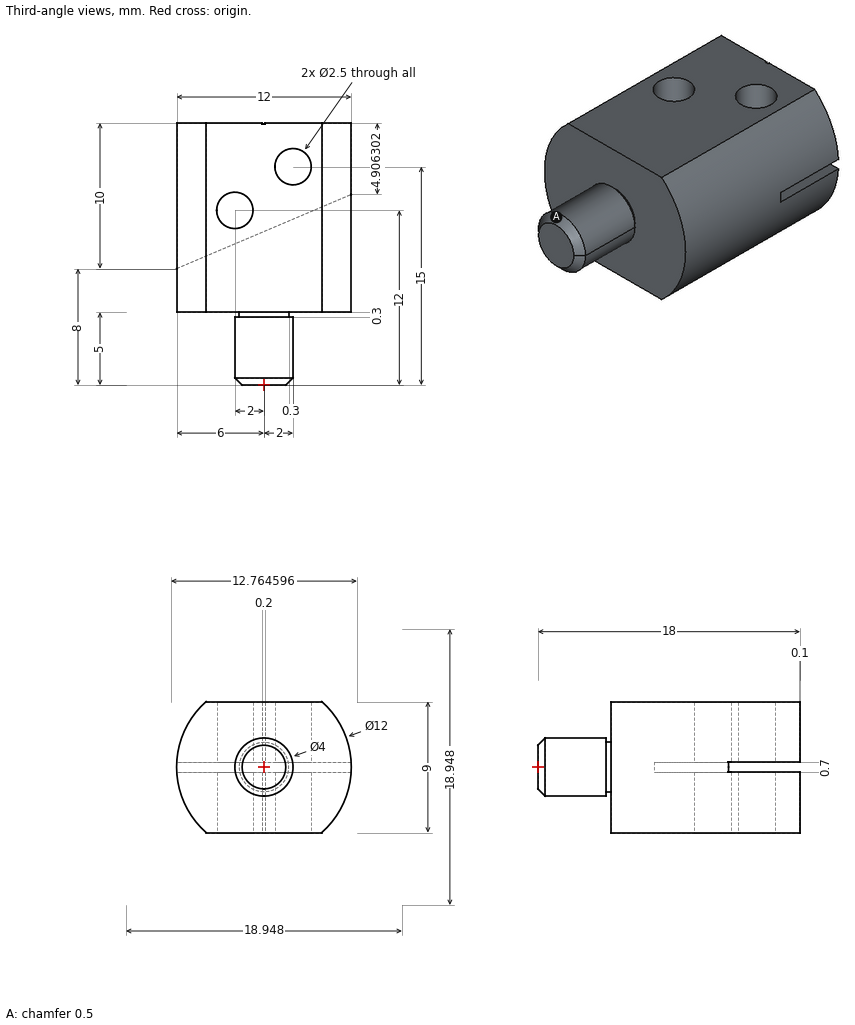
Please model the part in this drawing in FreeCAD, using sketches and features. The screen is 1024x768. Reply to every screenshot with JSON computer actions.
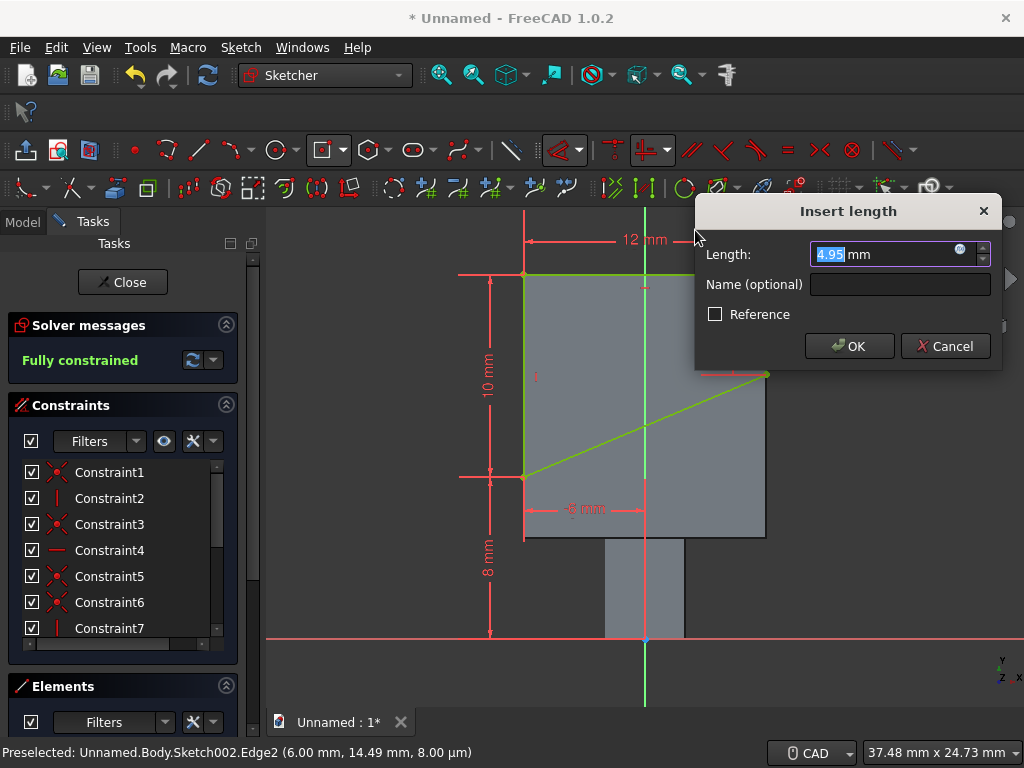
{"action": "type", "text": "4.906302"}
{"action": "key", "text": "Return"}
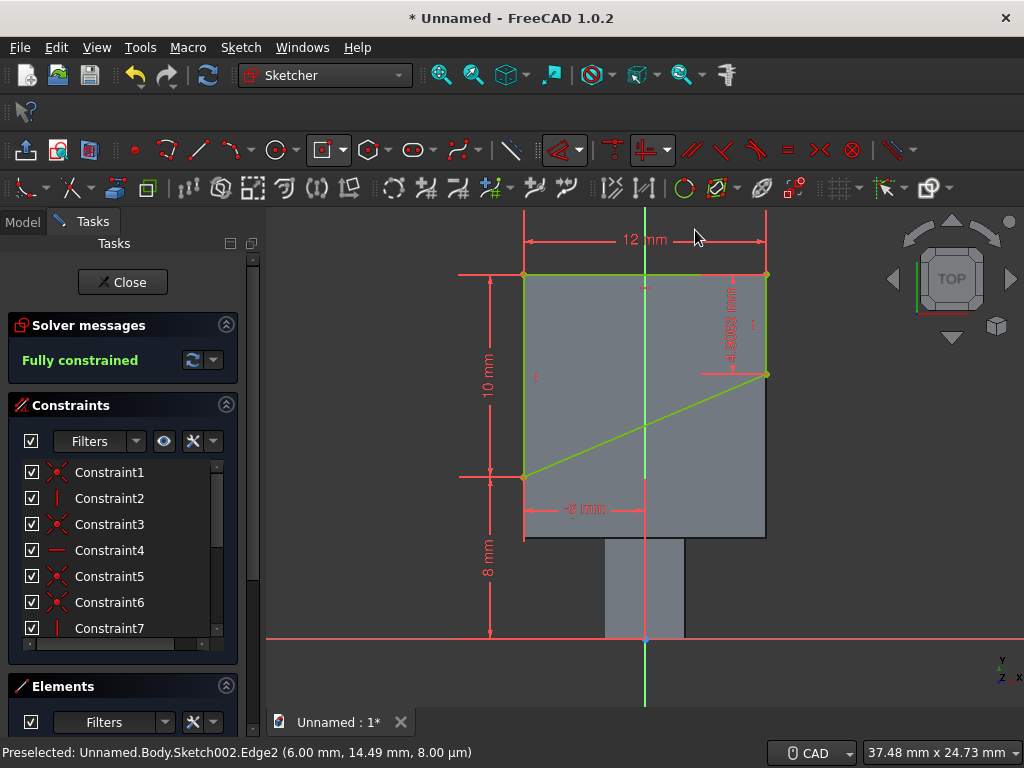
{"action": "left_click", "coordinate": [123, 282]}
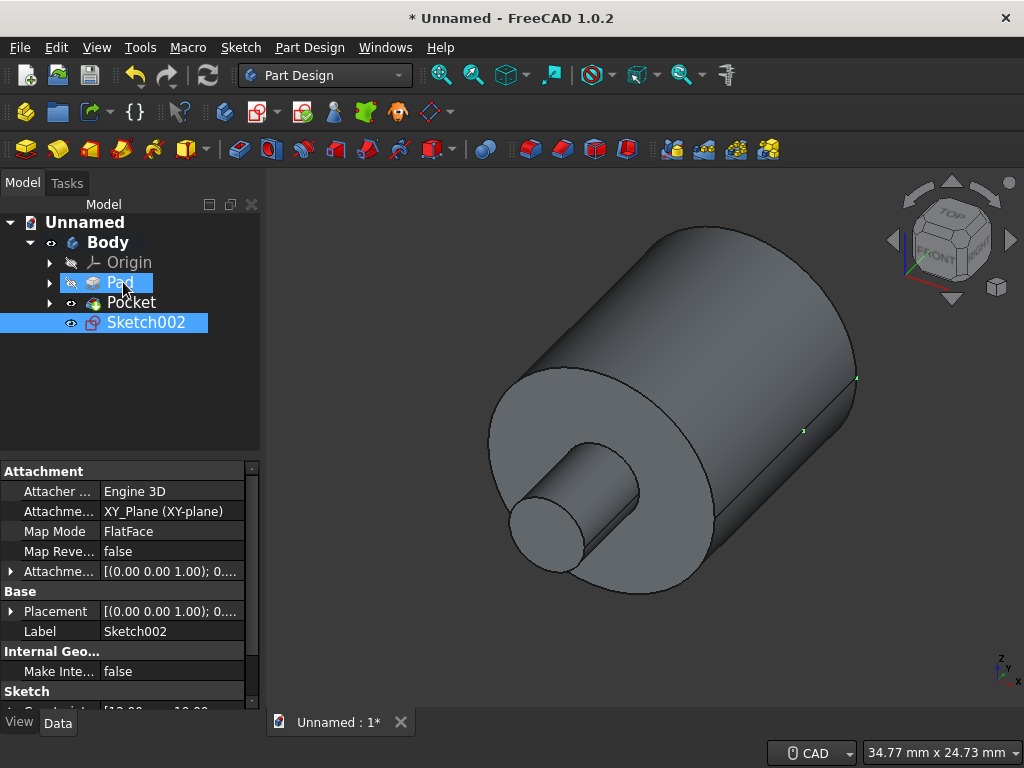
{"action": "left_click", "coordinate": [240, 150]}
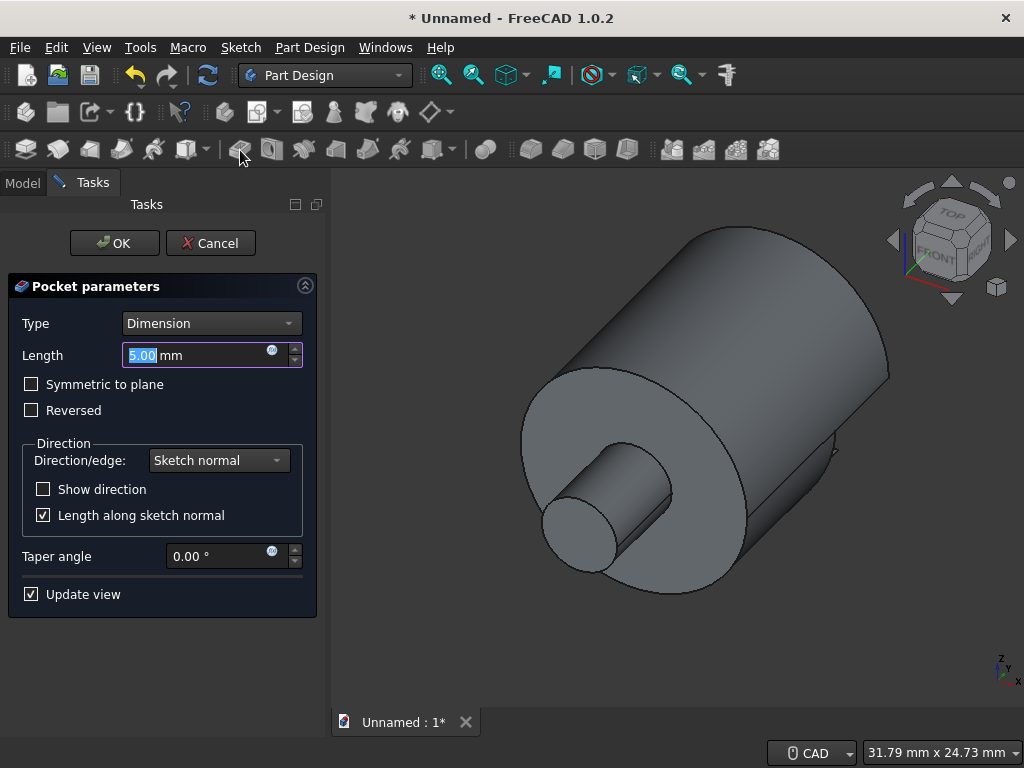
{"action": "type", "text": "0.7"}
{"action": "key", "text": "Tab"}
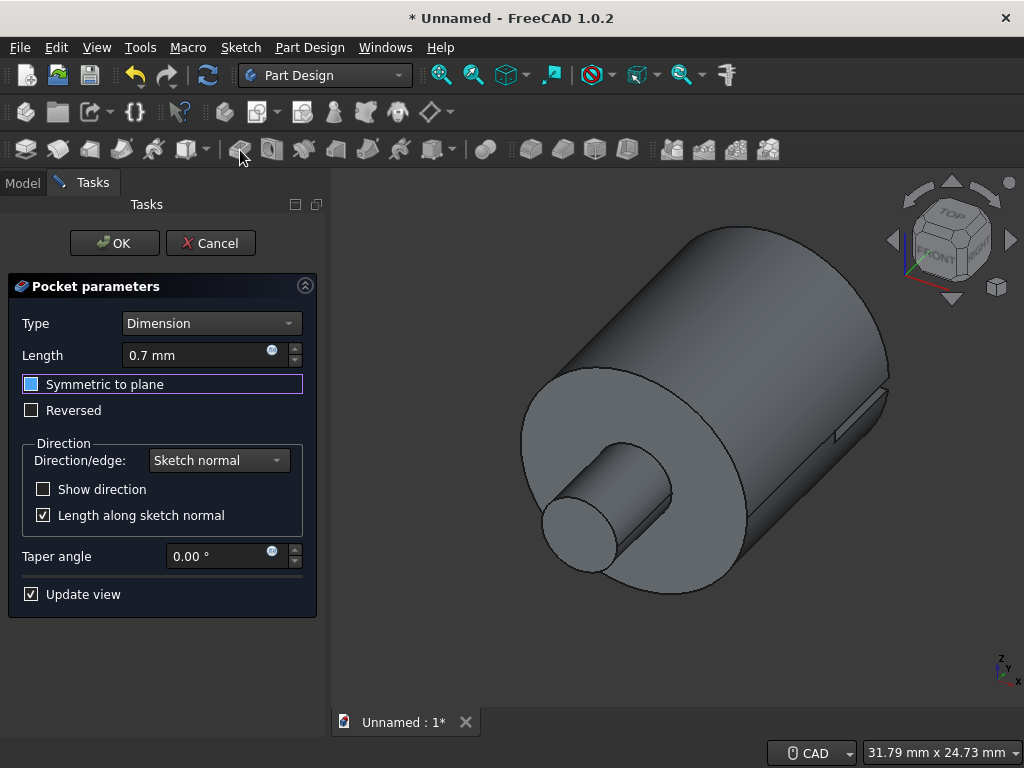
{"action": "left_click", "coordinate": [30, 384]}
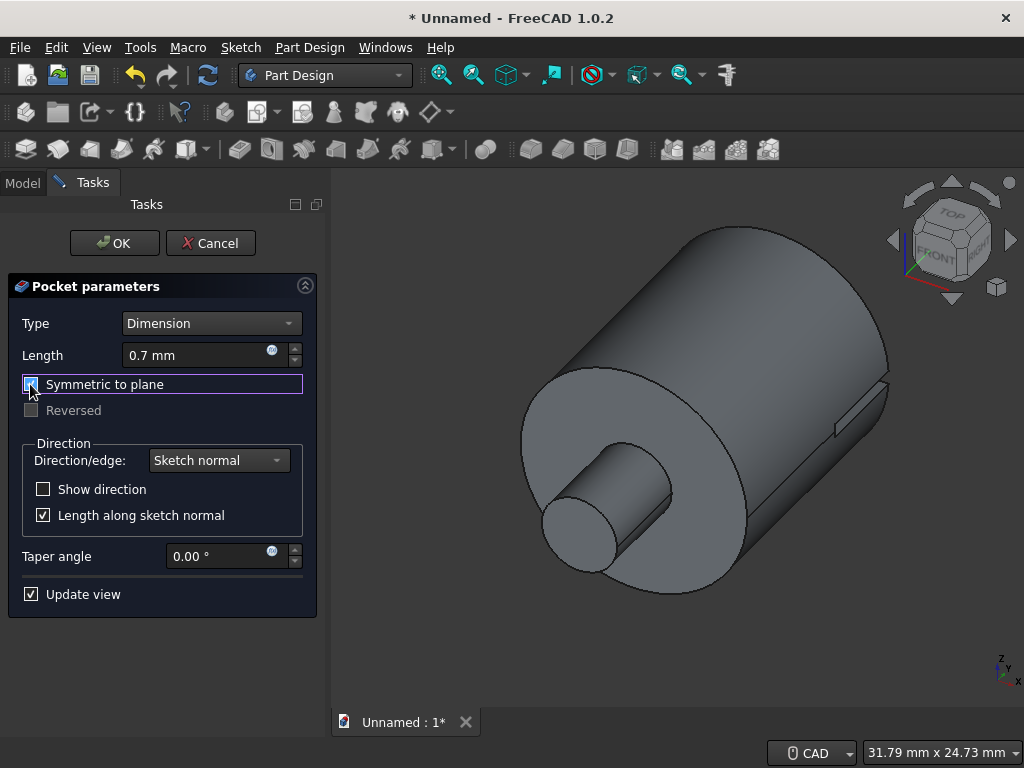
{"action": "left_click", "coordinate": [115, 243]}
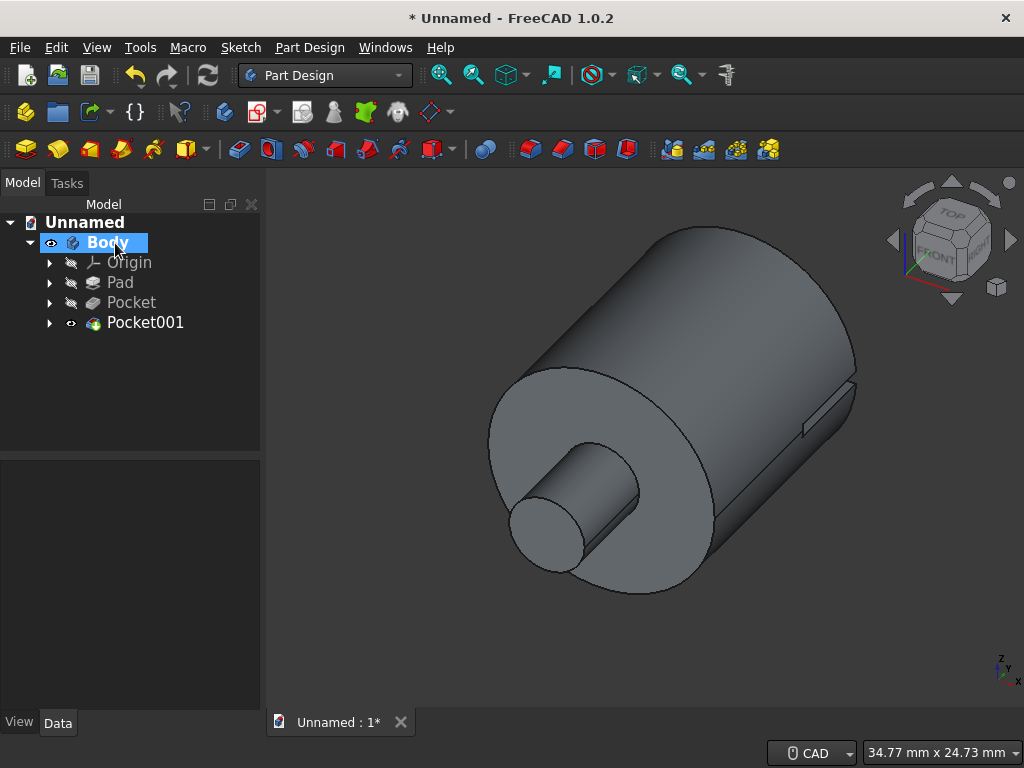
{"action": "left_click", "coordinate": [516, 503]}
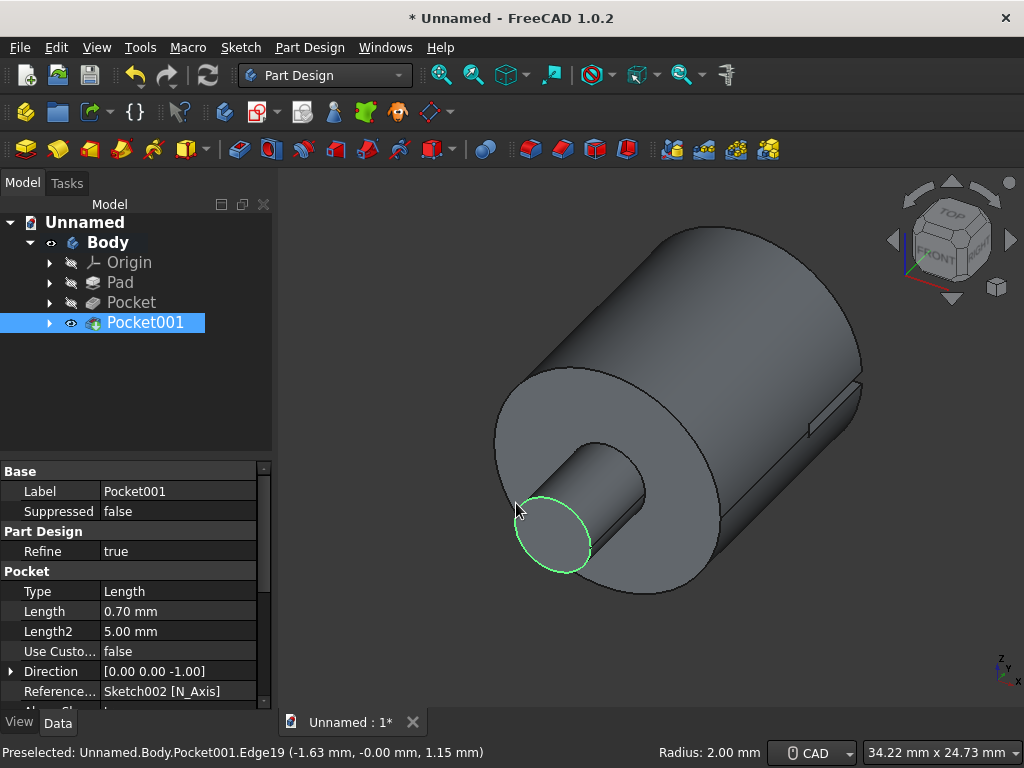
{"action": "left_click", "coordinate": [564, 150]}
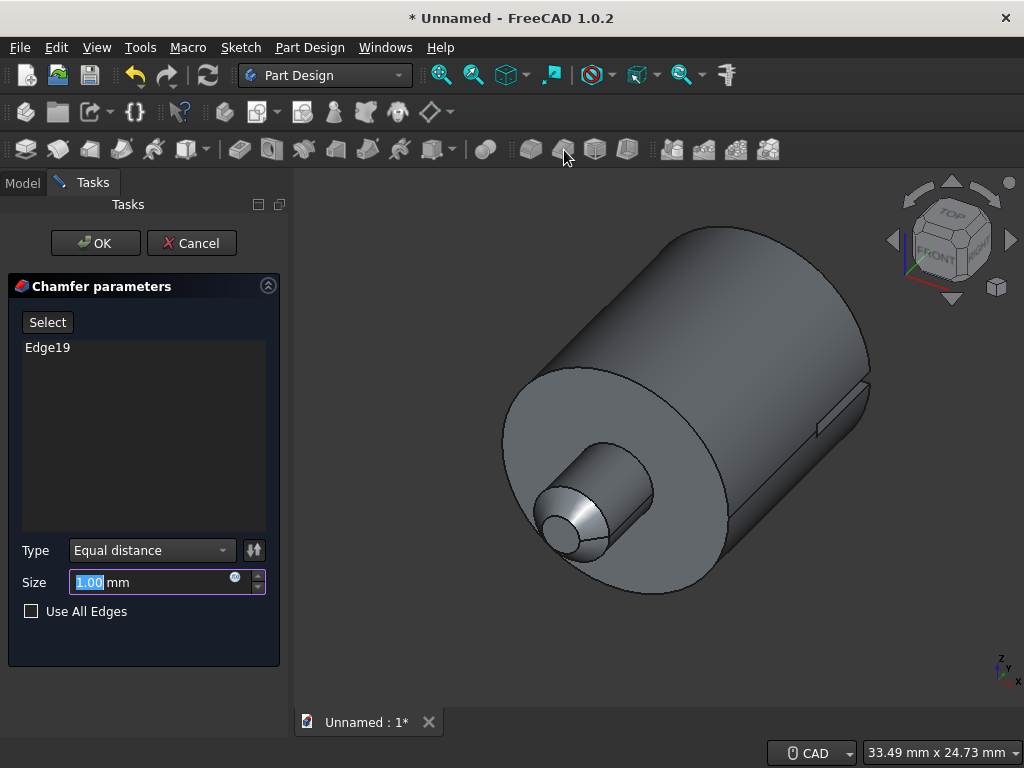
{"action": "type", "text": "0.5"}
{"action": "key", "text": "Tab"}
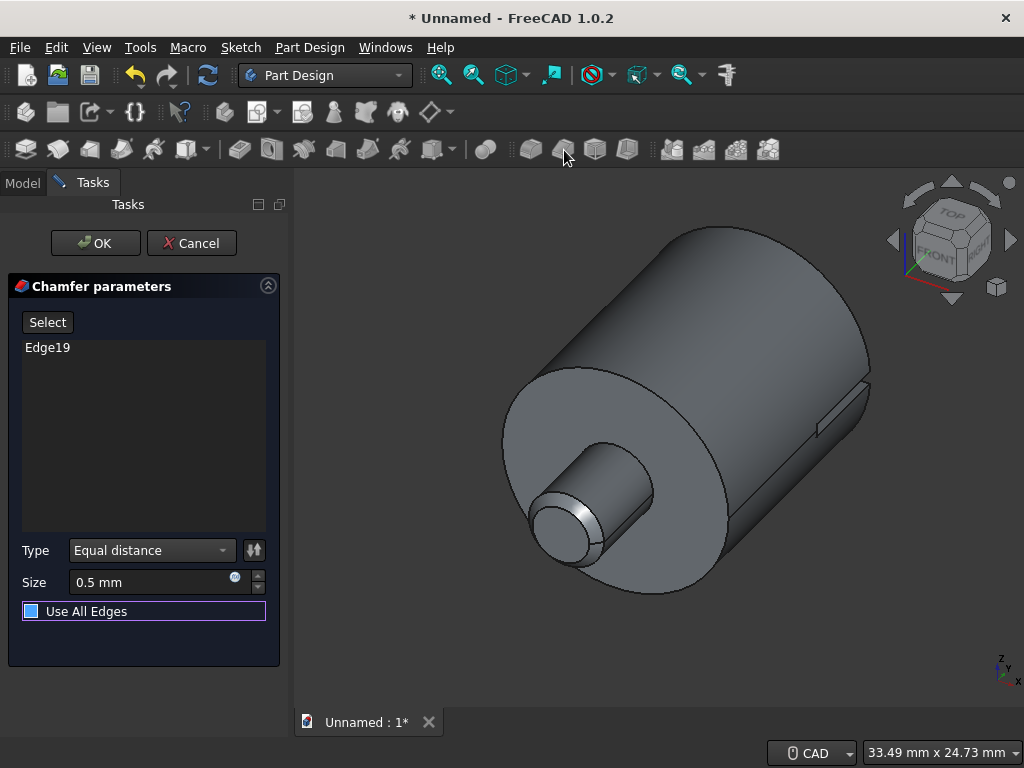
{"action": "left_click", "coordinate": [96, 243]}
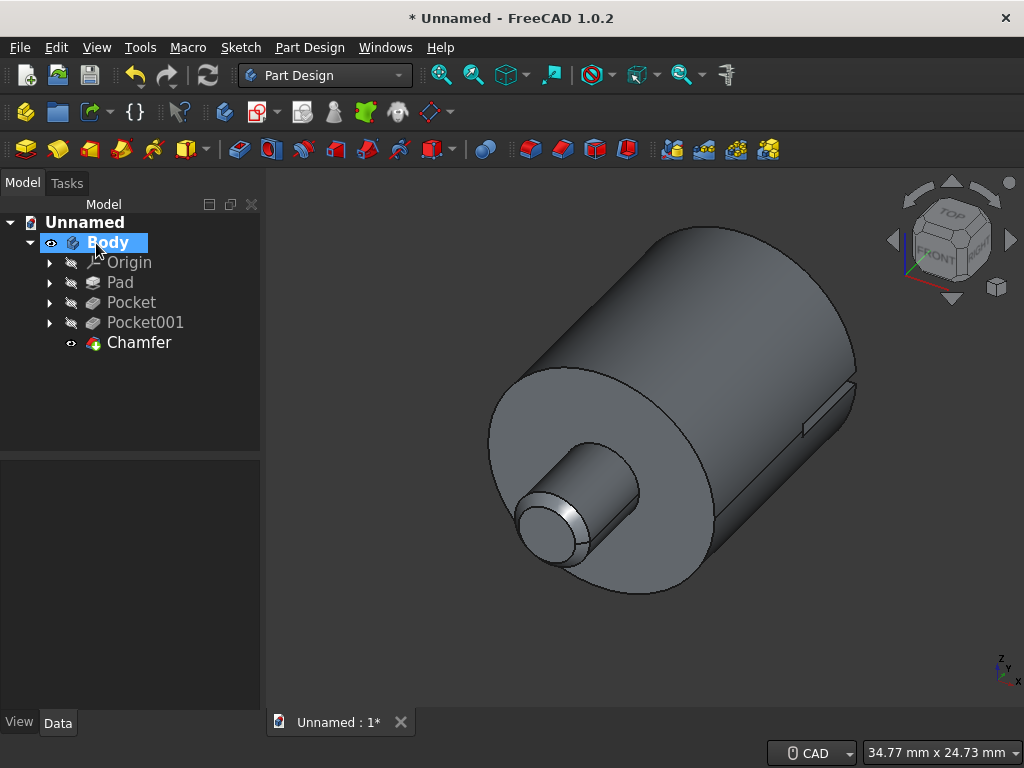
{"action": "left_click", "coordinate": [258, 112]}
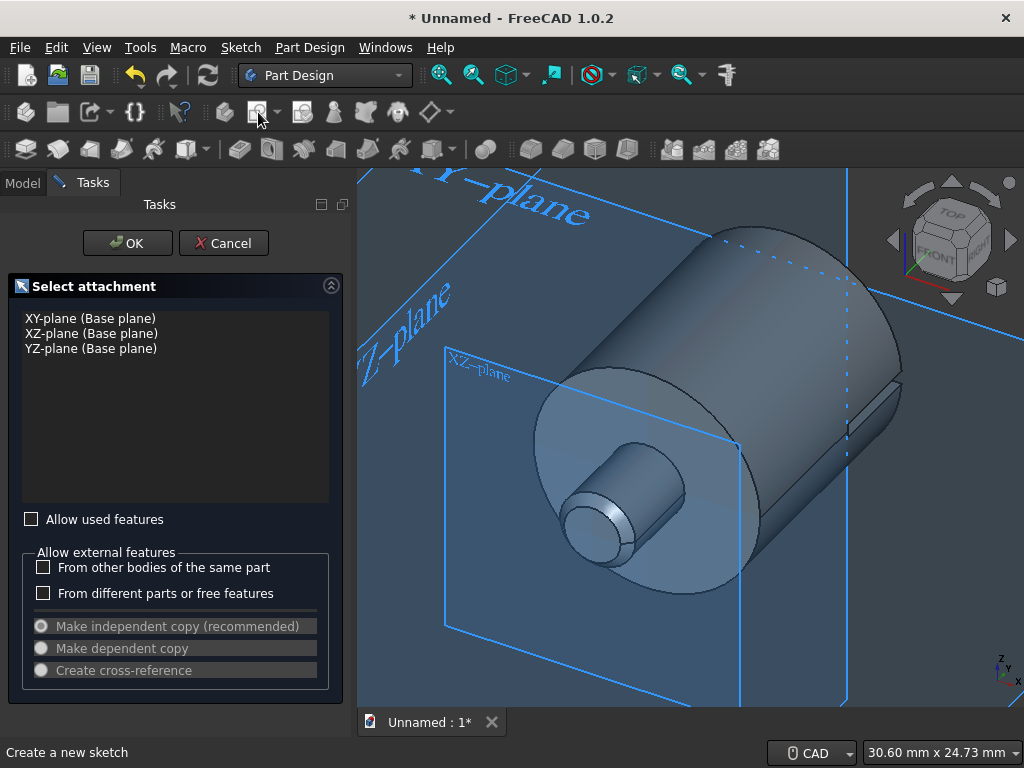
{"action": "left_click", "coordinate": [82, 318]}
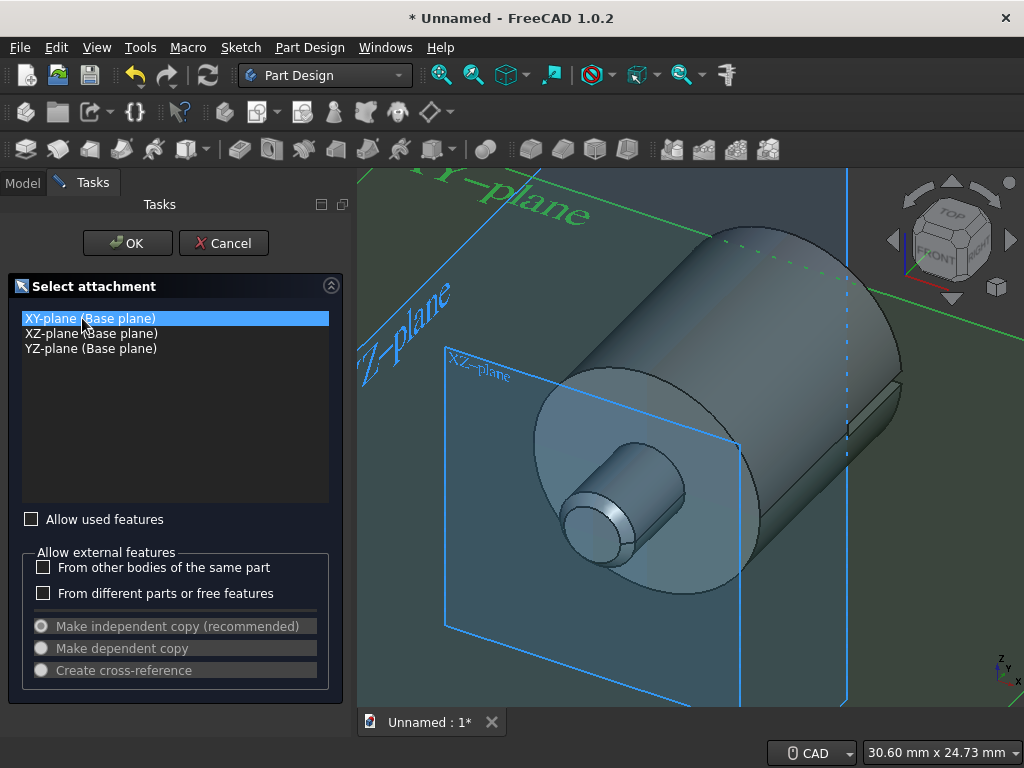
{"action": "left_click", "coordinate": [128, 243]}